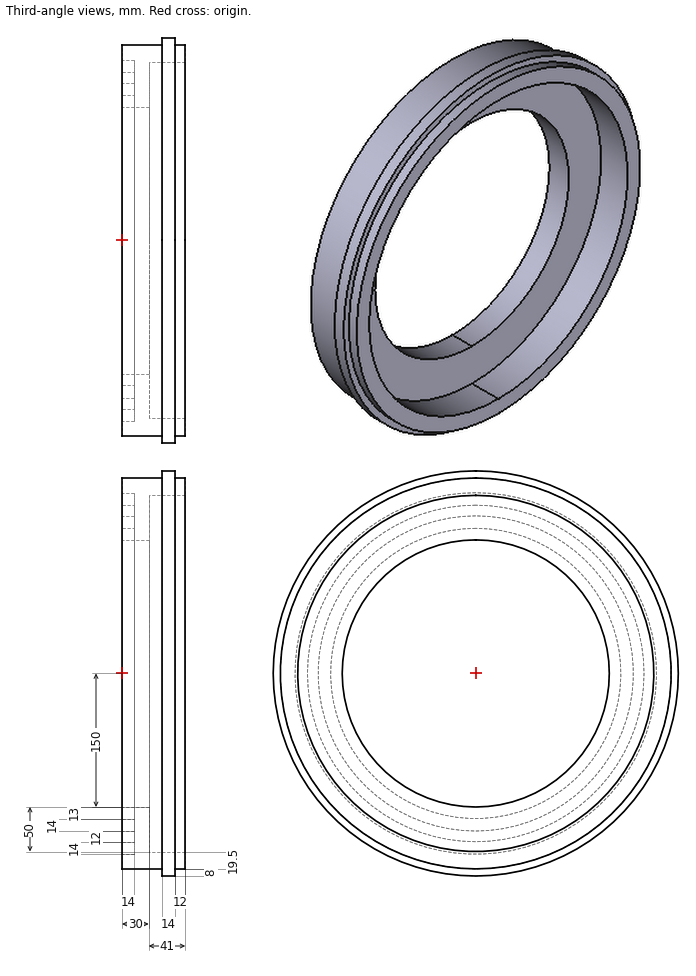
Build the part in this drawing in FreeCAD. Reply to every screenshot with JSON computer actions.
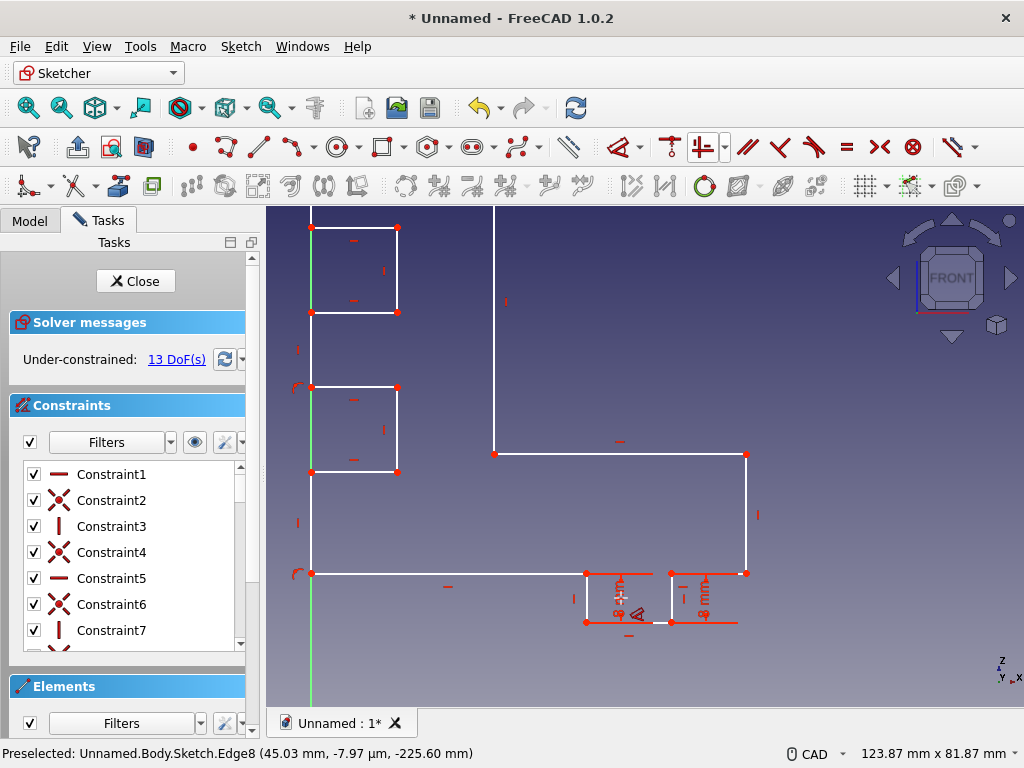
{"action": "scroll", "coordinate": [674, 605], "scroll_direction": "down", "scroll_amount": 2}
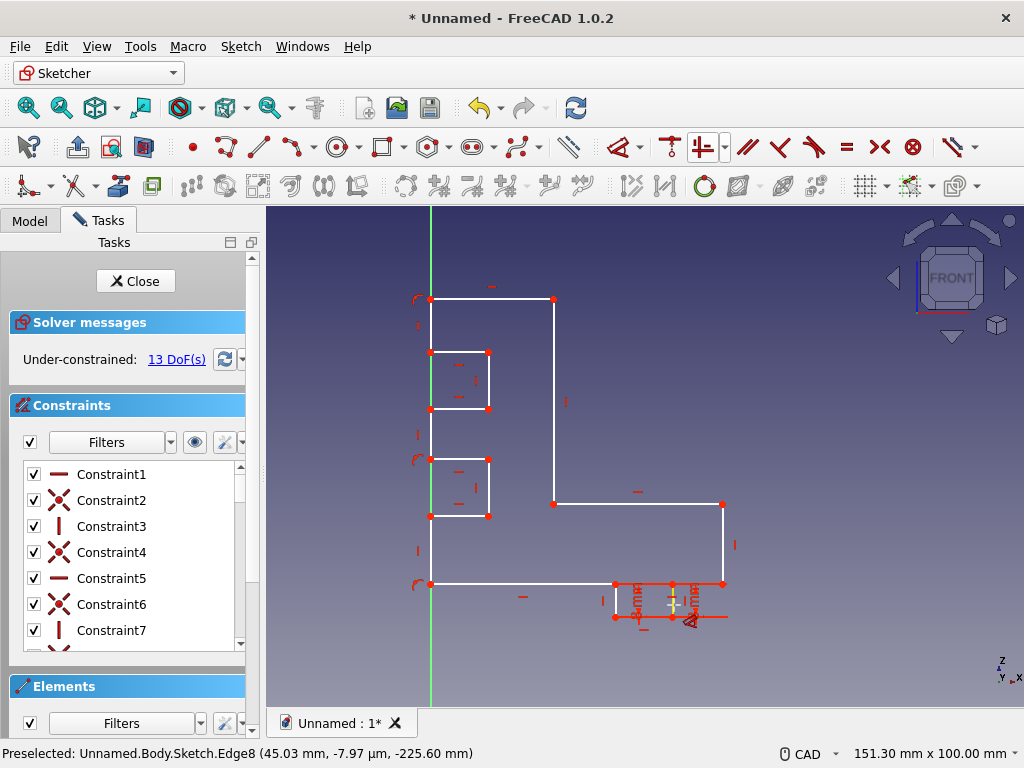
{"action": "left_click", "coordinate": [468, 299]}
{"action": "left_click", "coordinate": [492, 265]}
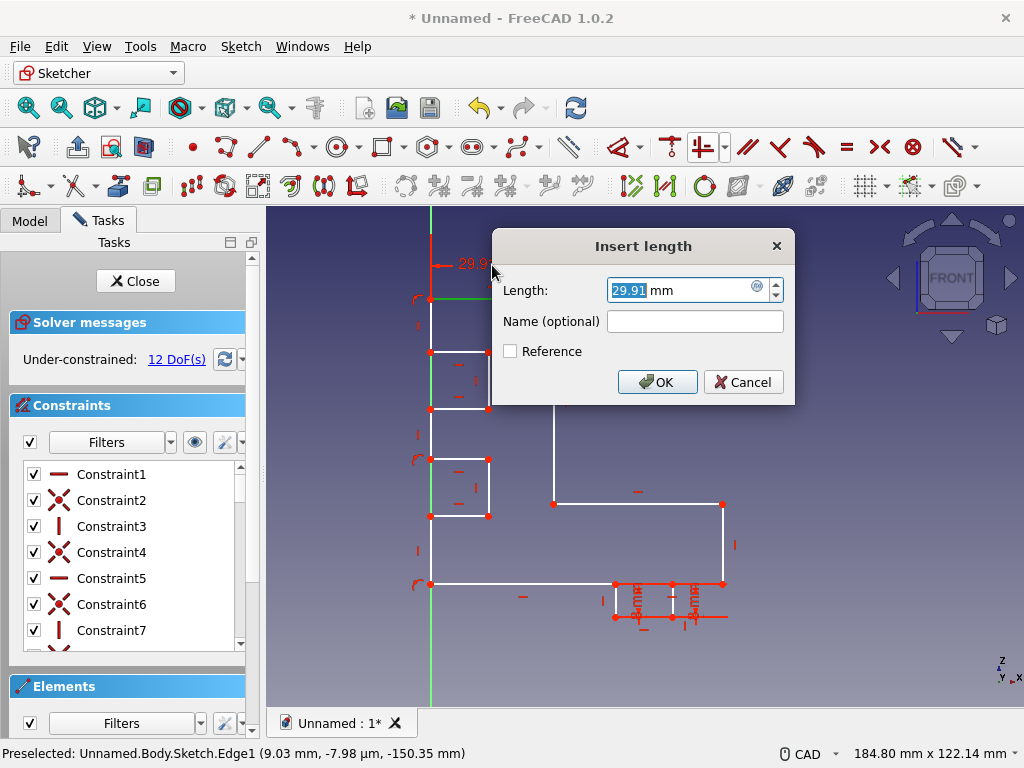
{"action": "type", "text": "30"}
{"action": "key", "text": "Return"}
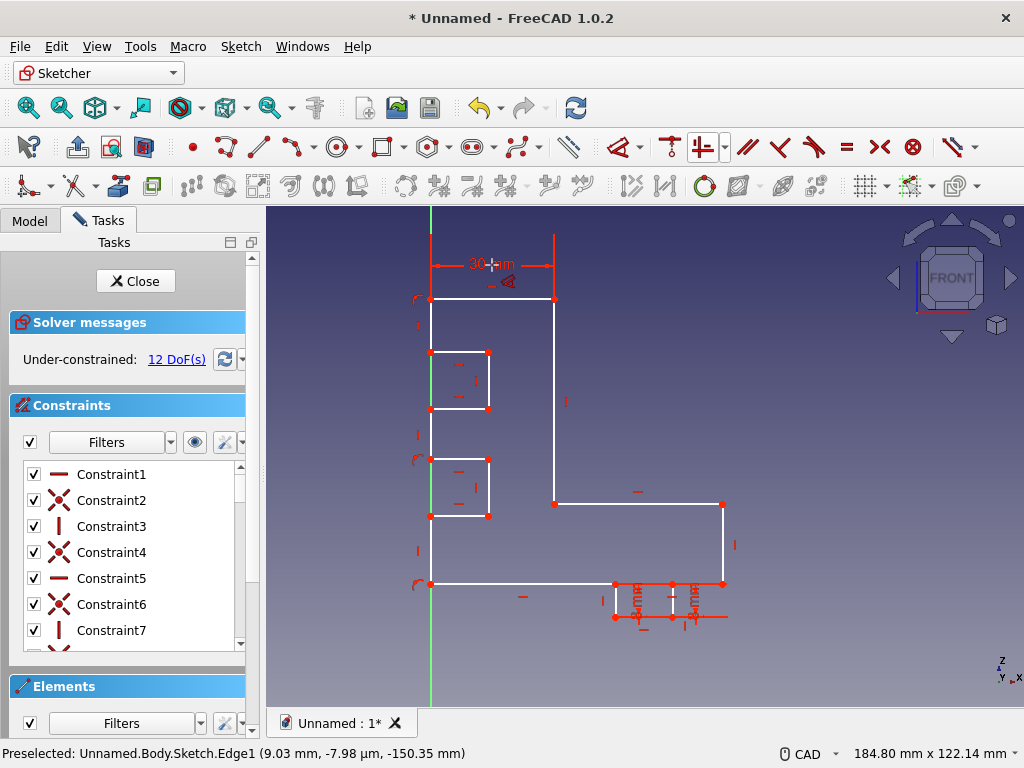
{"action": "left_click", "coordinate": [554, 361]}
{"action": "left_click", "coordinate": [520, 402]}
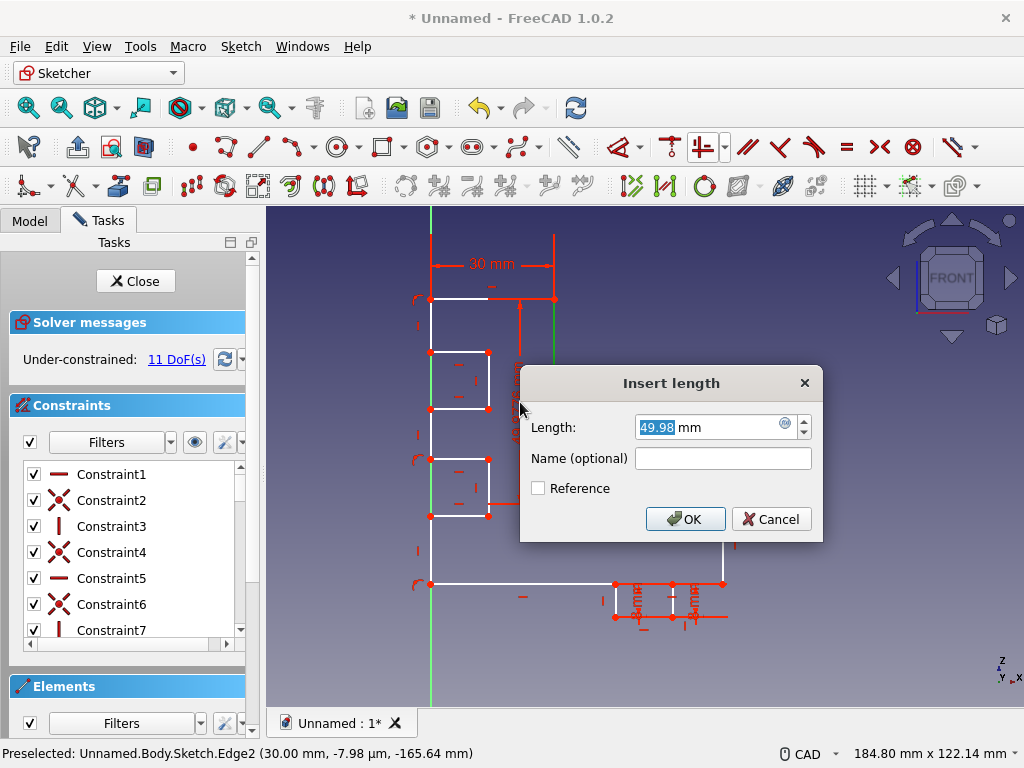
{"action": "type", "text": "50"}
{"action": "key", "text": "Return"}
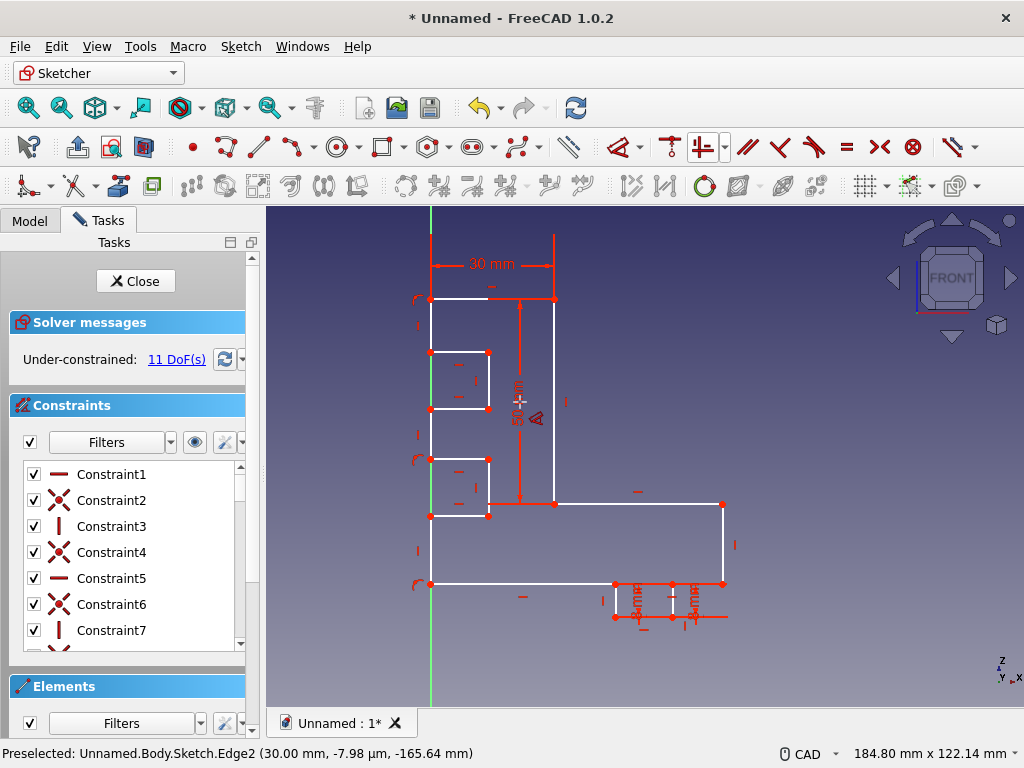
{"action": "left_click", "coordinate": [605, 504]}
{"action": "left_click", "coordinate": [638, 538]}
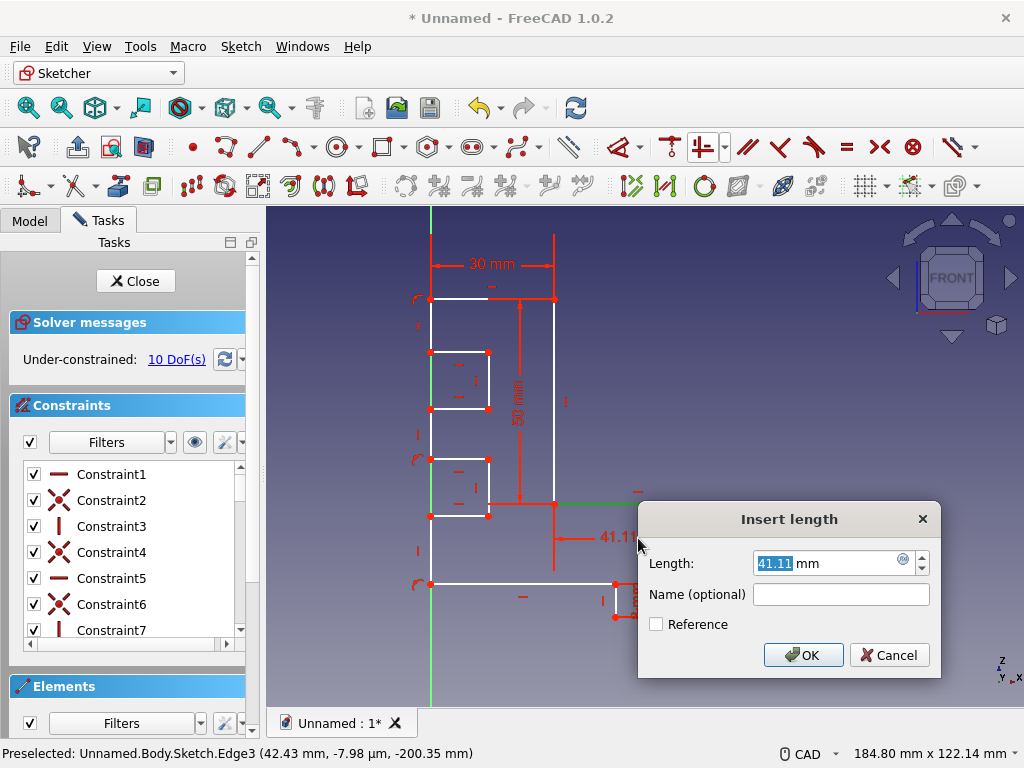
{"action": "type", "text": "41"}
{"action": "key", "text": "Return"}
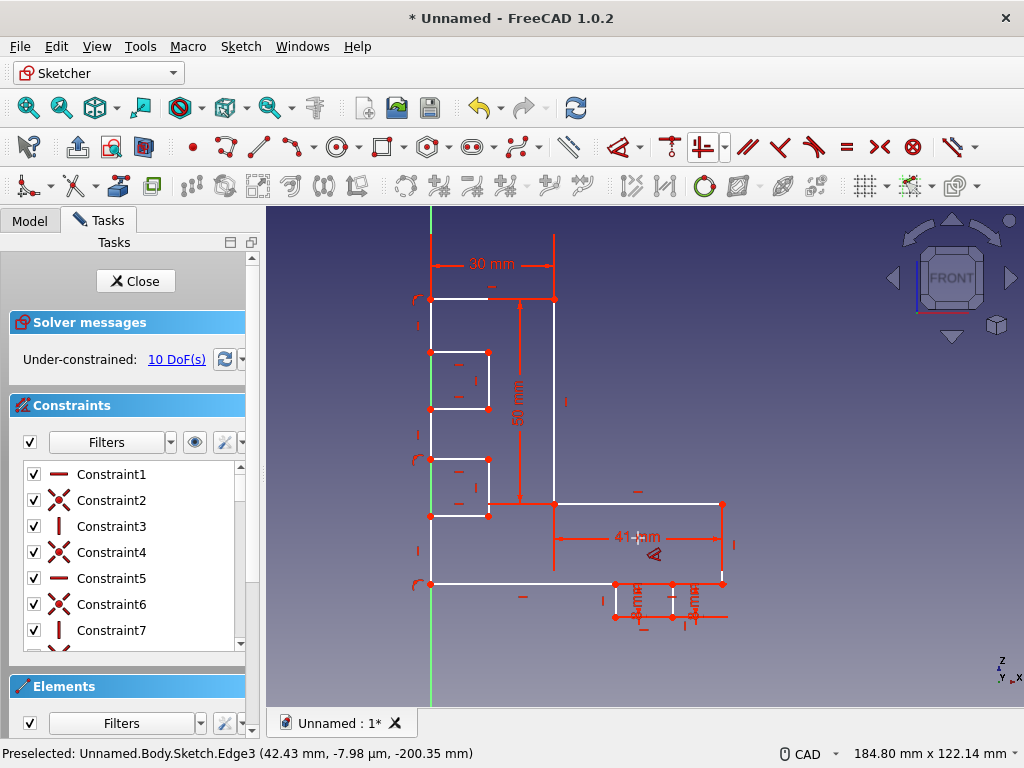
{"action": "left_click", "coordinate": [707, 584]}
{"action": "left_click", "coordinate": [709, 550]}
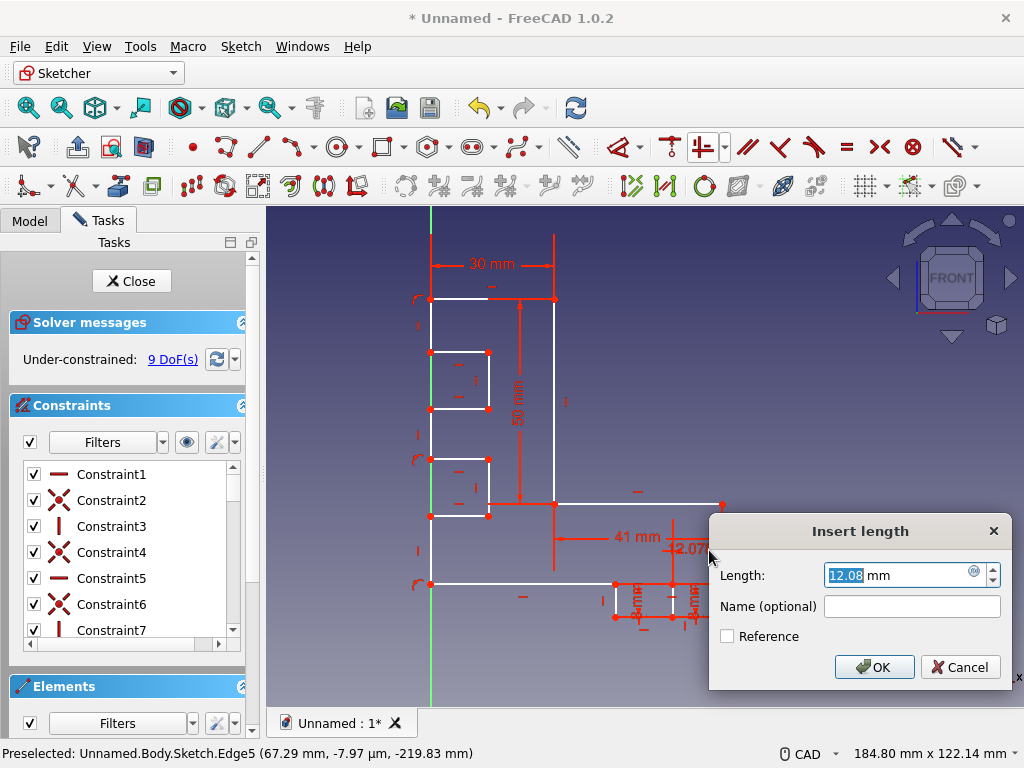
{"action": "type", "text": "12"}
{"action": "key", "text": "Return"}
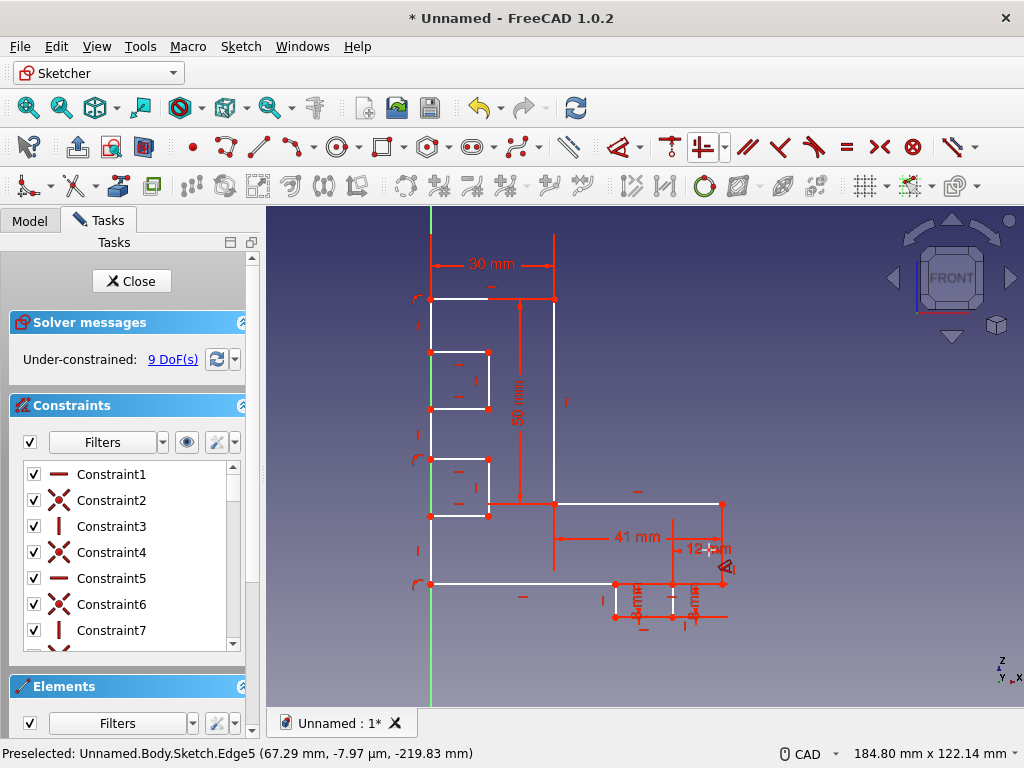
{"action": "left_click", "coordinate": [656, 617]}
{"action": "left_click", "coordinate": [644, 651]}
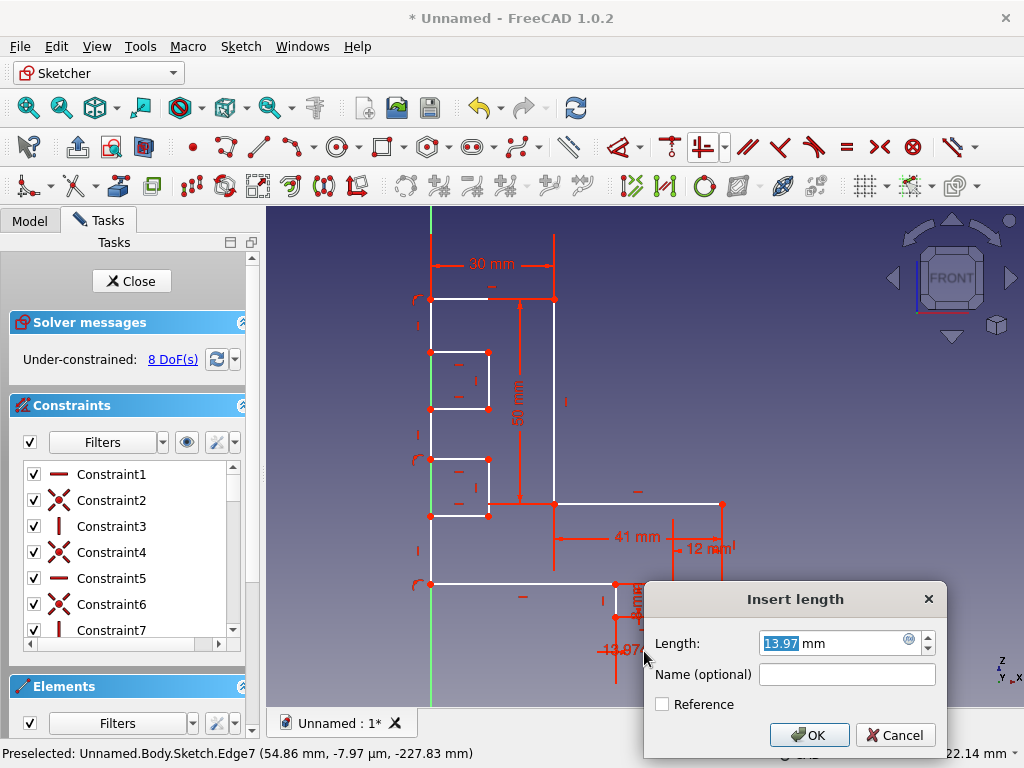
{"action": "type", "text": "14"}
{"action": "key", "text": "Return"}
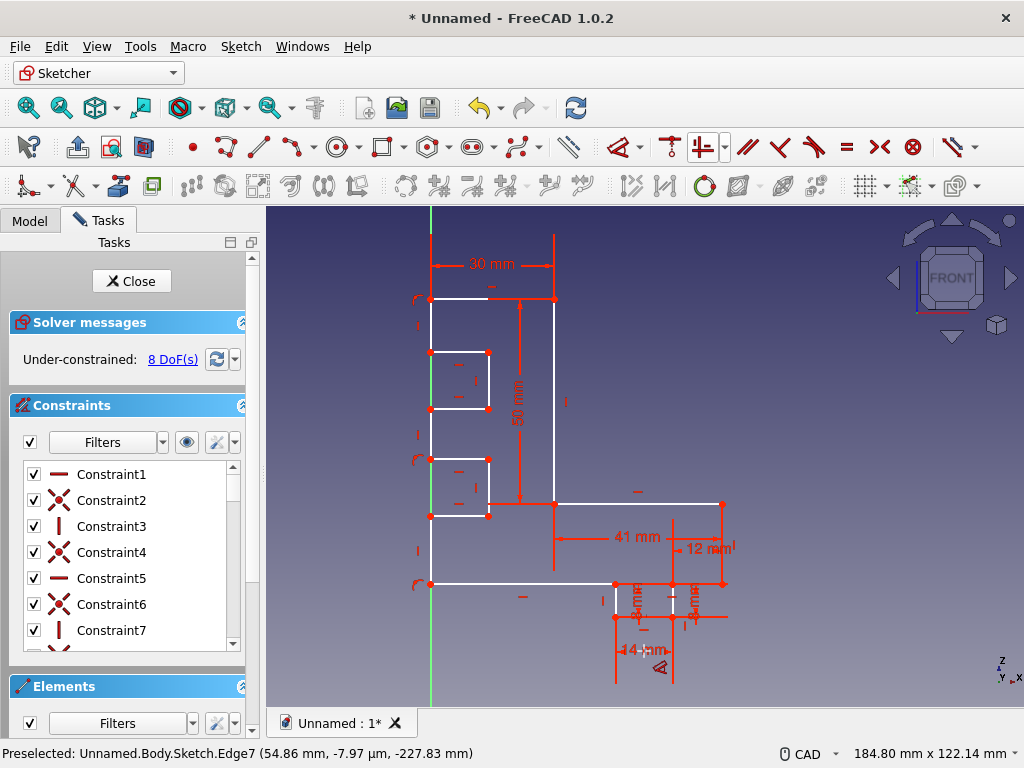
{"action": "left_click", "coordinate": [448, 516]}
{"action": "left_click", "coordinate": [460, 550]}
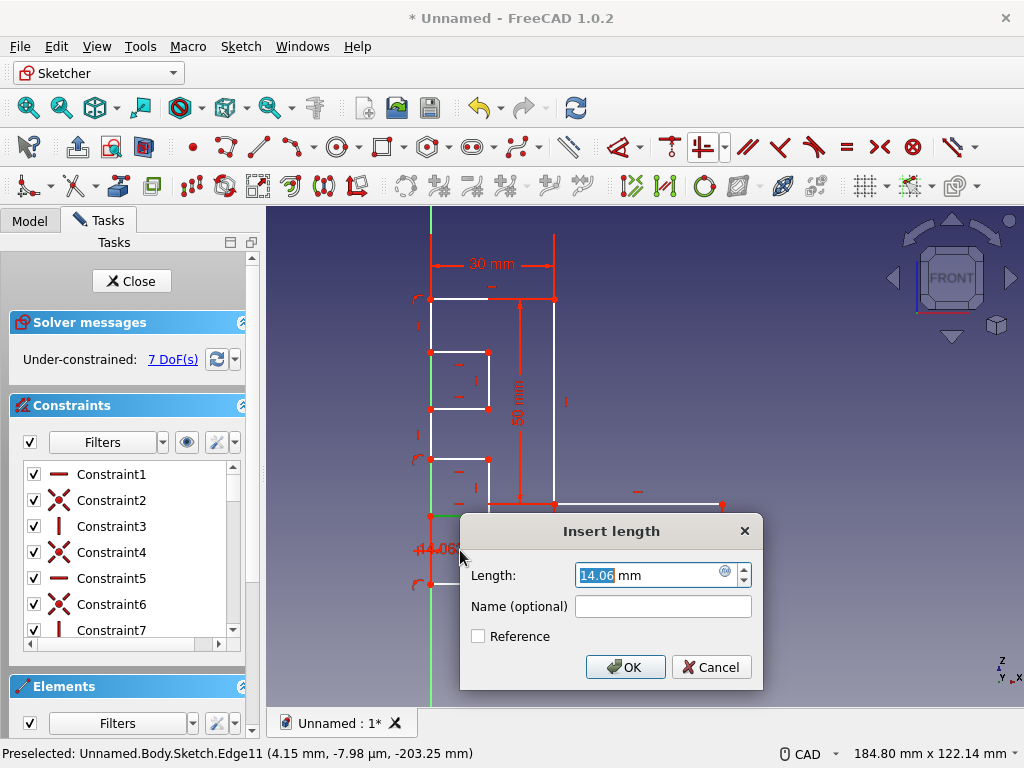
{"action": "type", "text": "14"}
{"action": "key", "text": "Return"}